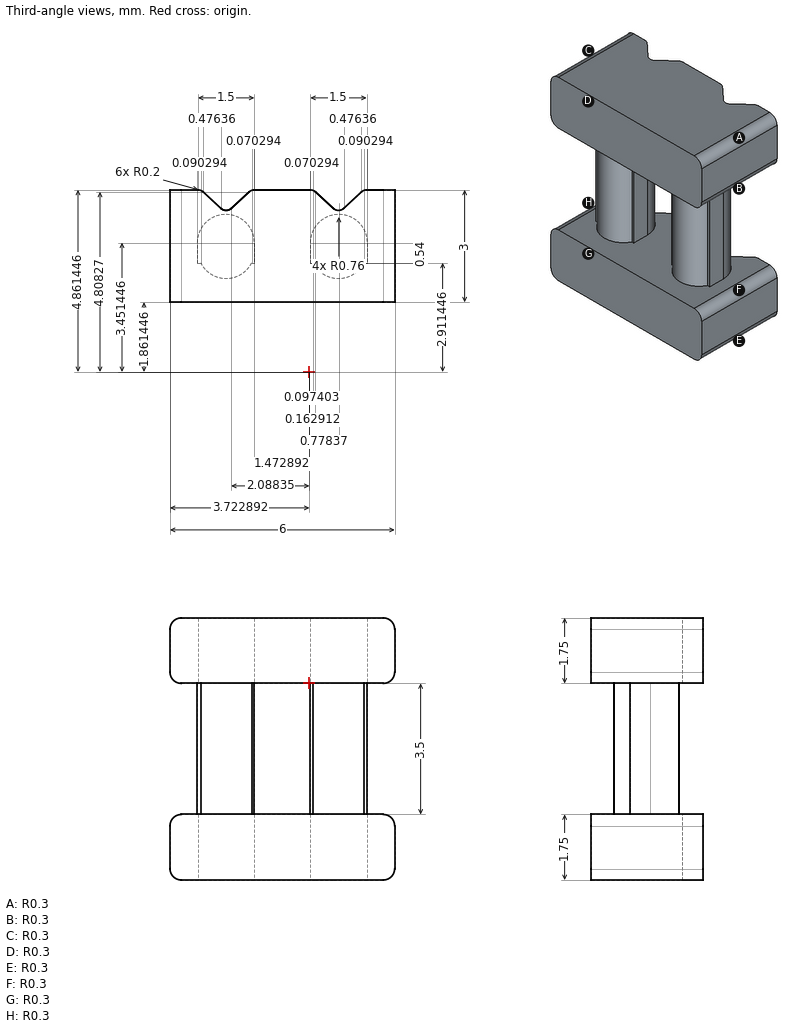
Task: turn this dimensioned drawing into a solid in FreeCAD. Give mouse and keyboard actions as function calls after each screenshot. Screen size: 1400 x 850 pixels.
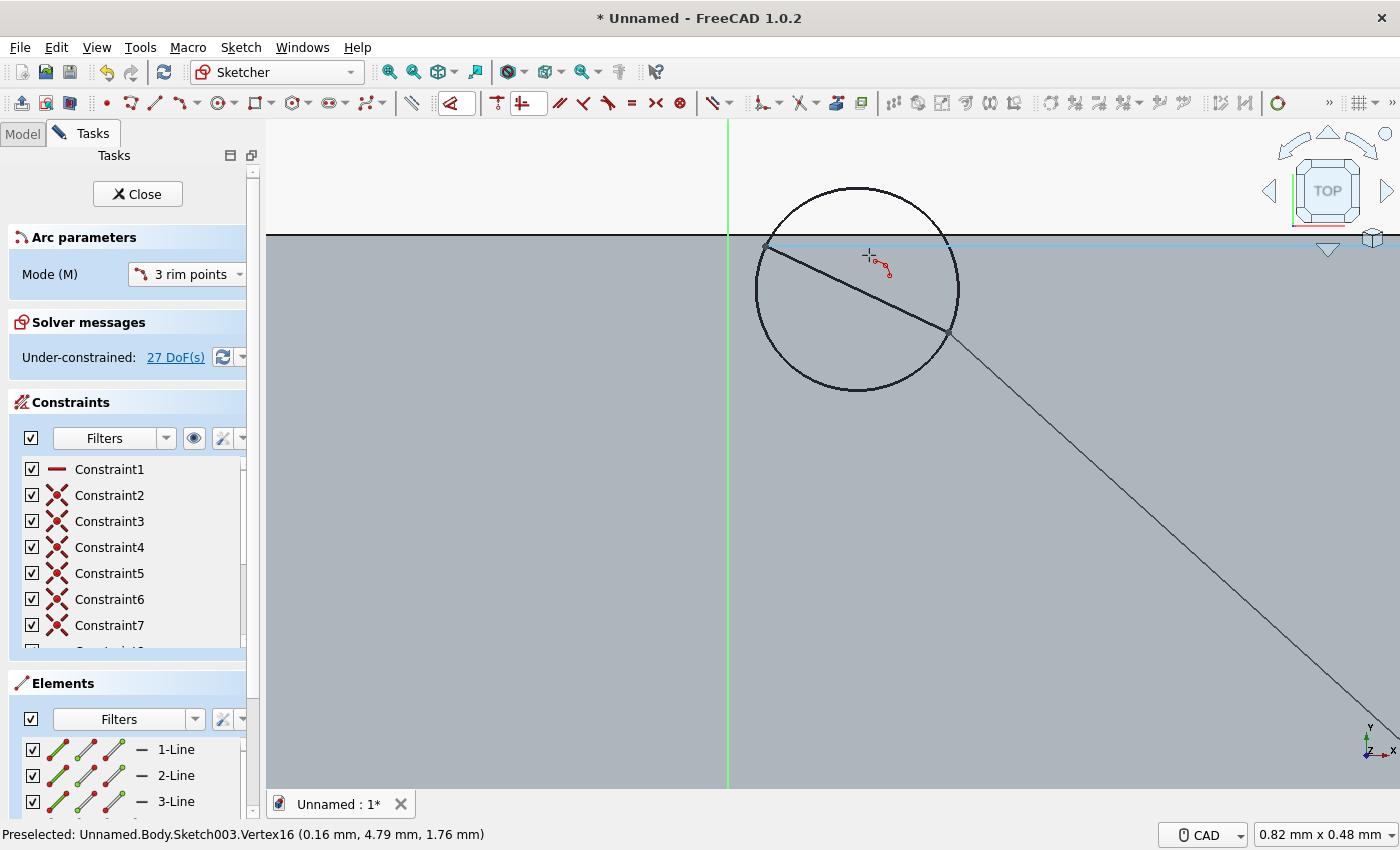
click(867, 254)
key(Escape)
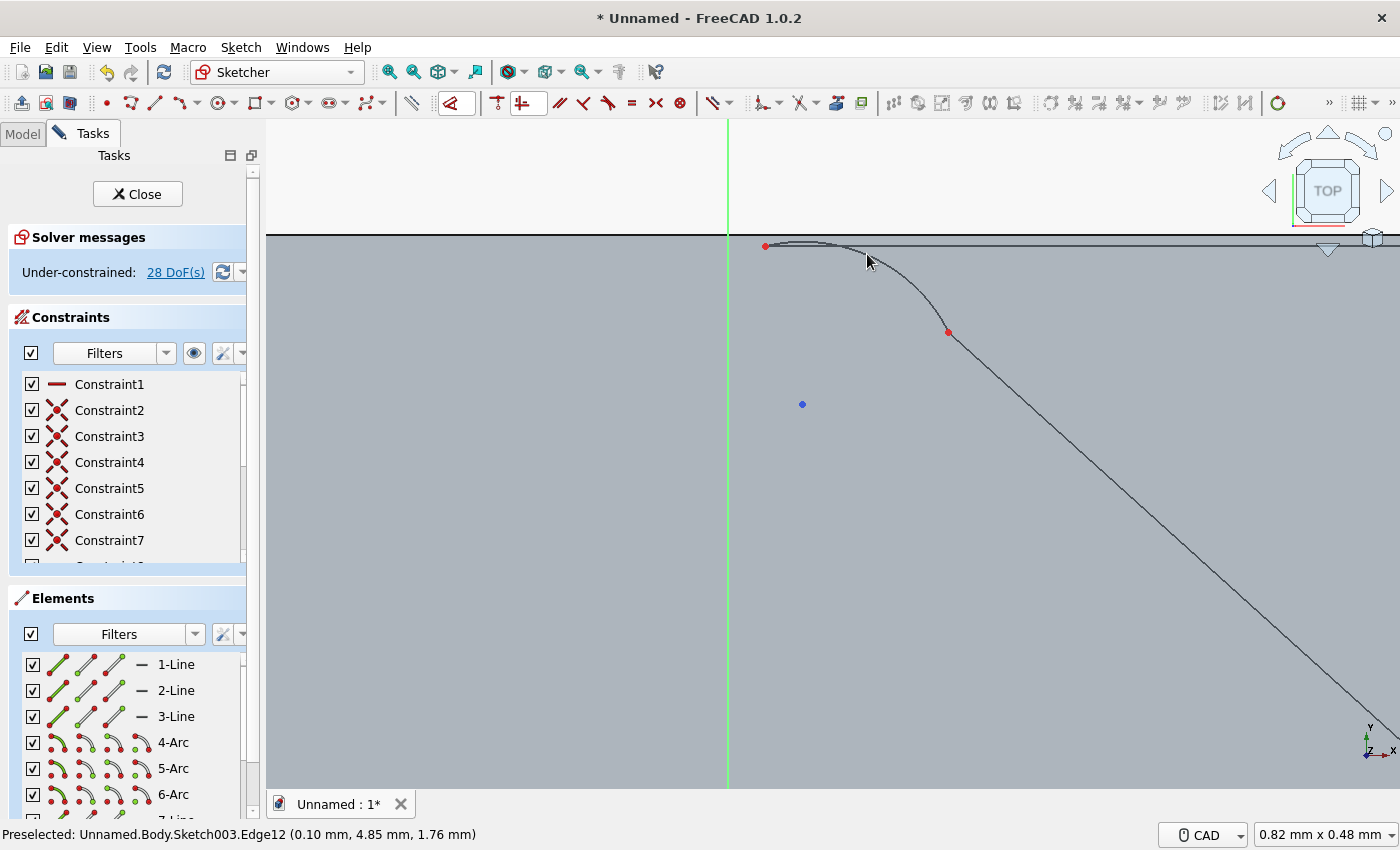
scroll(832, 250, down, 14)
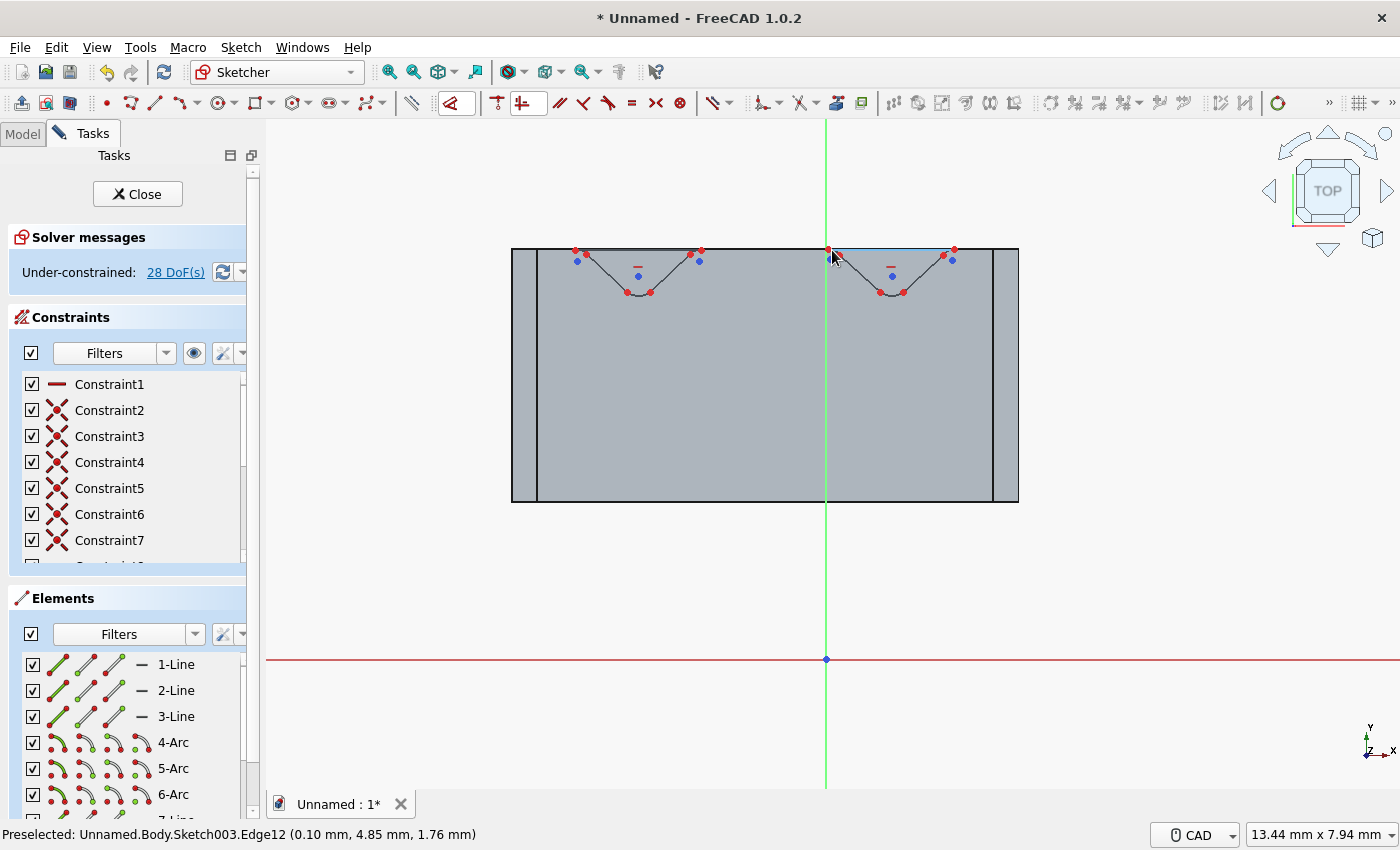
click(664, 250)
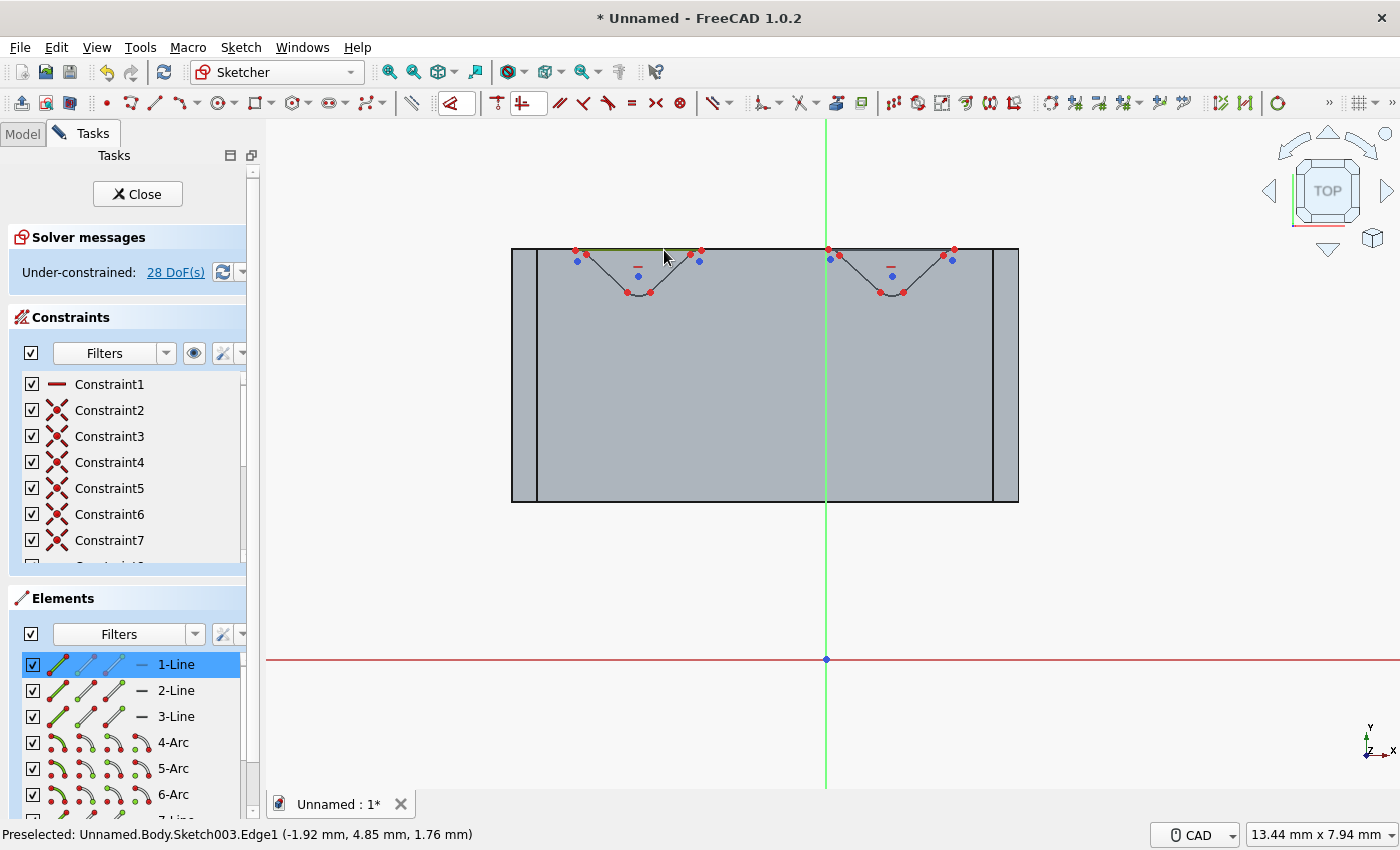
scroll(585, 252, up, 9)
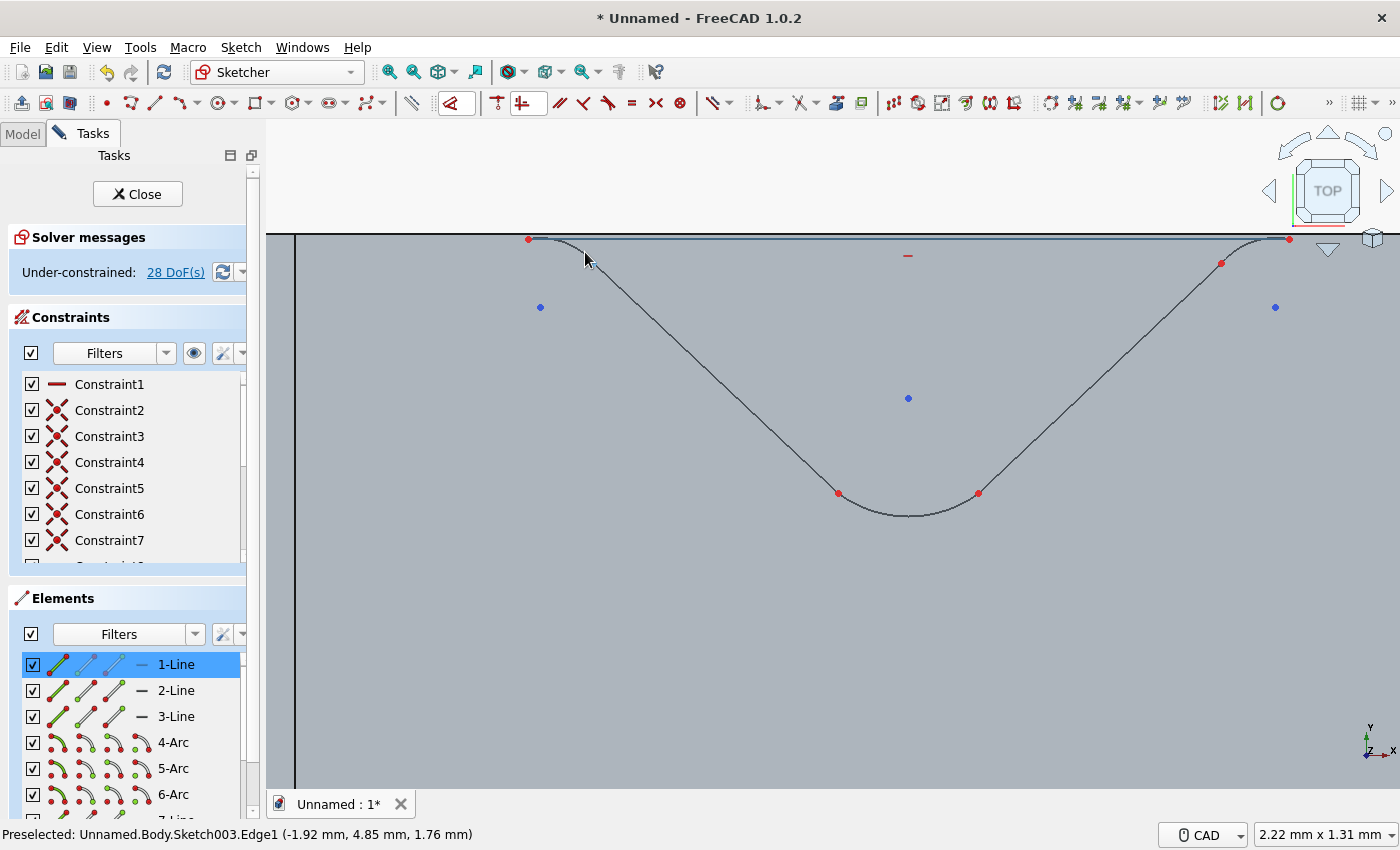
click(583, 253)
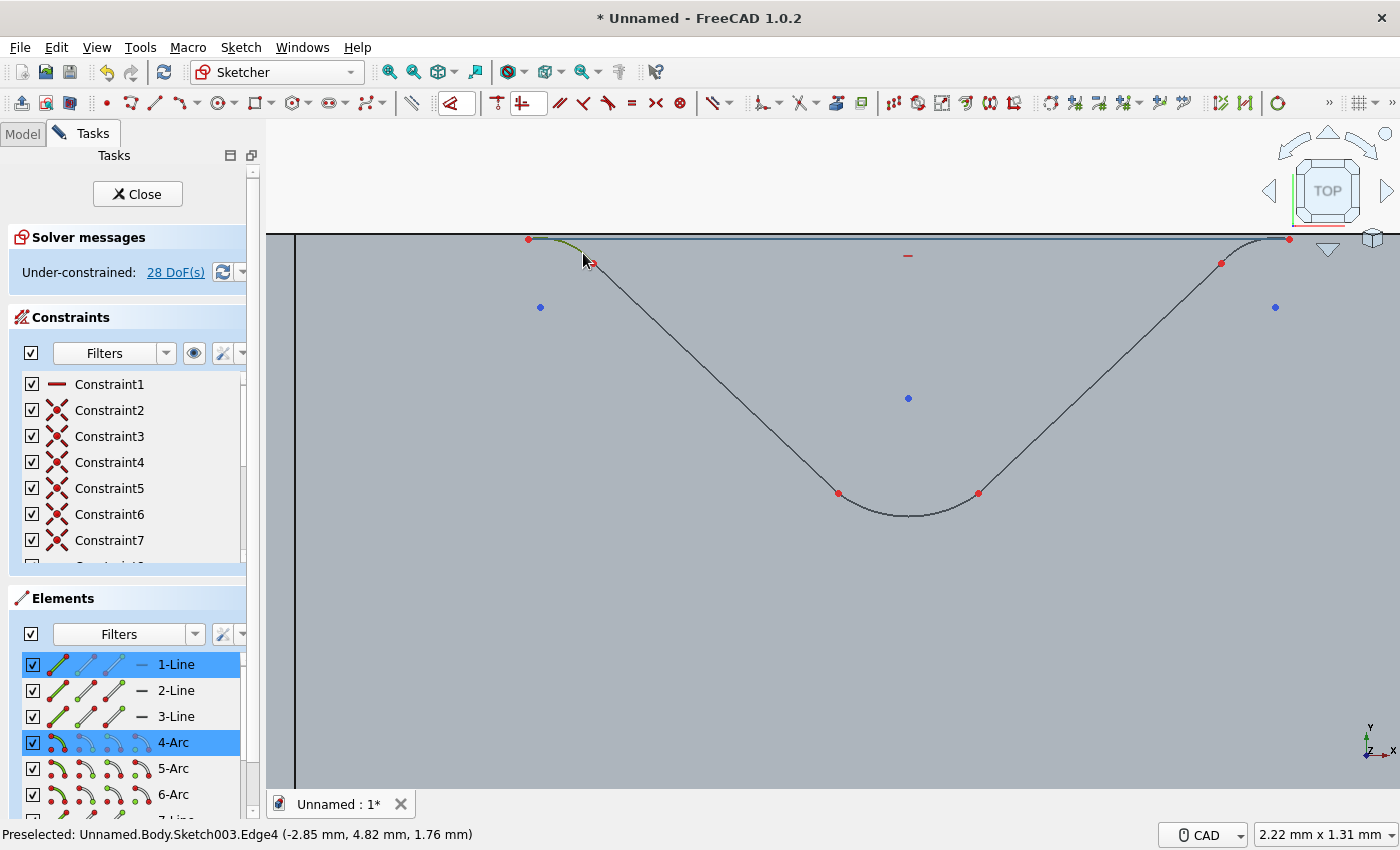
click(608, 104)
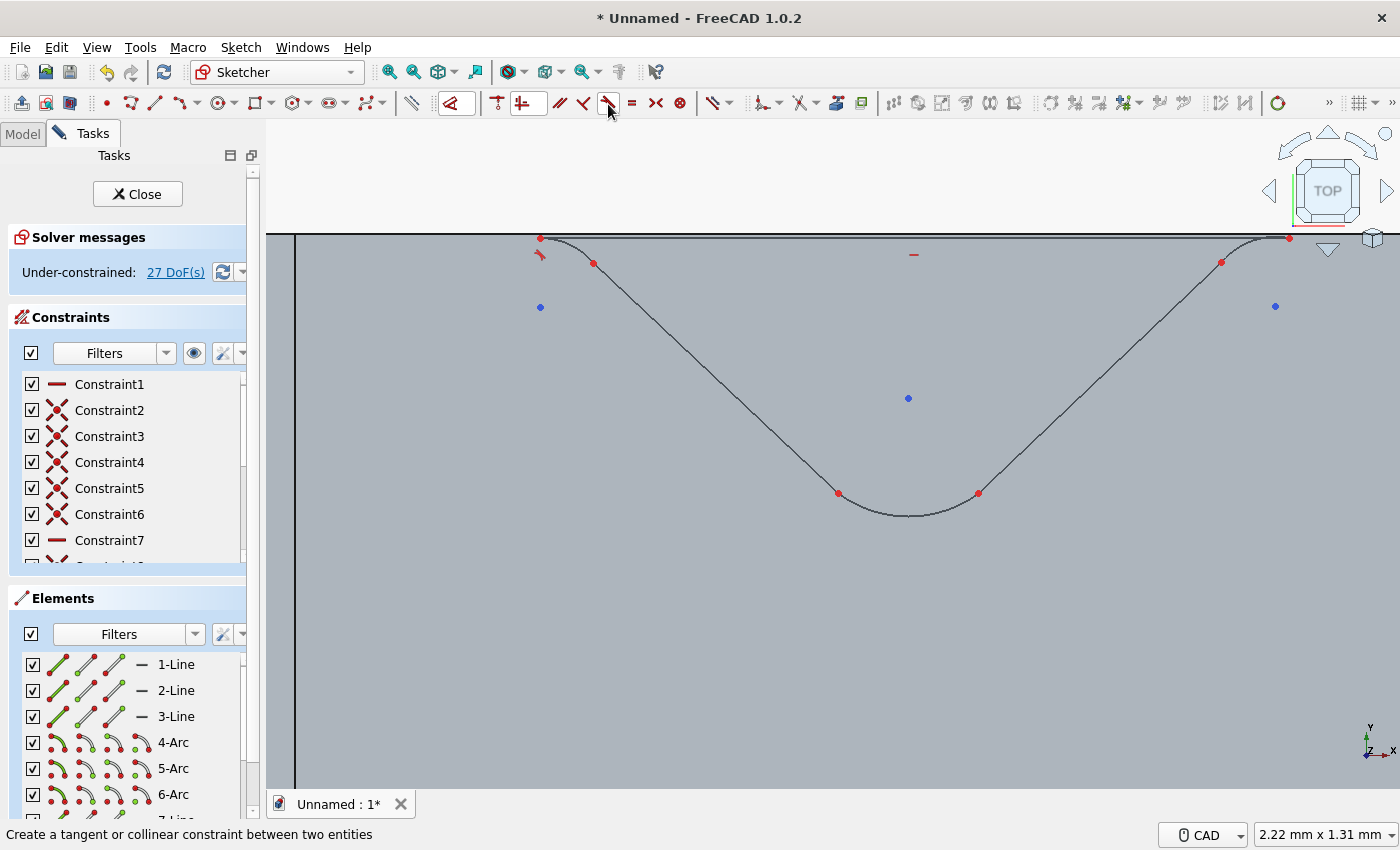
scroll(584, 252, down, 9)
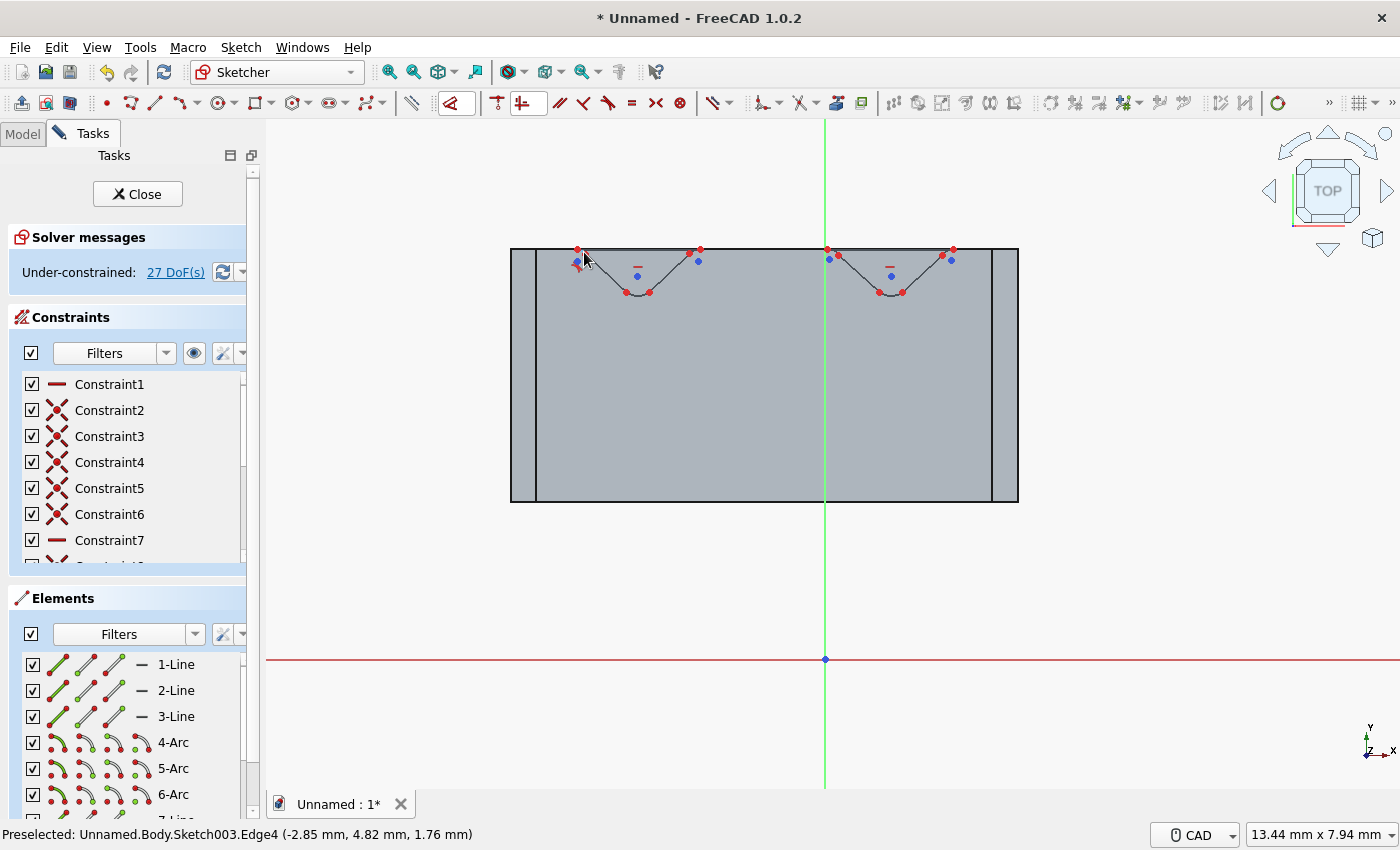
click(664, 250)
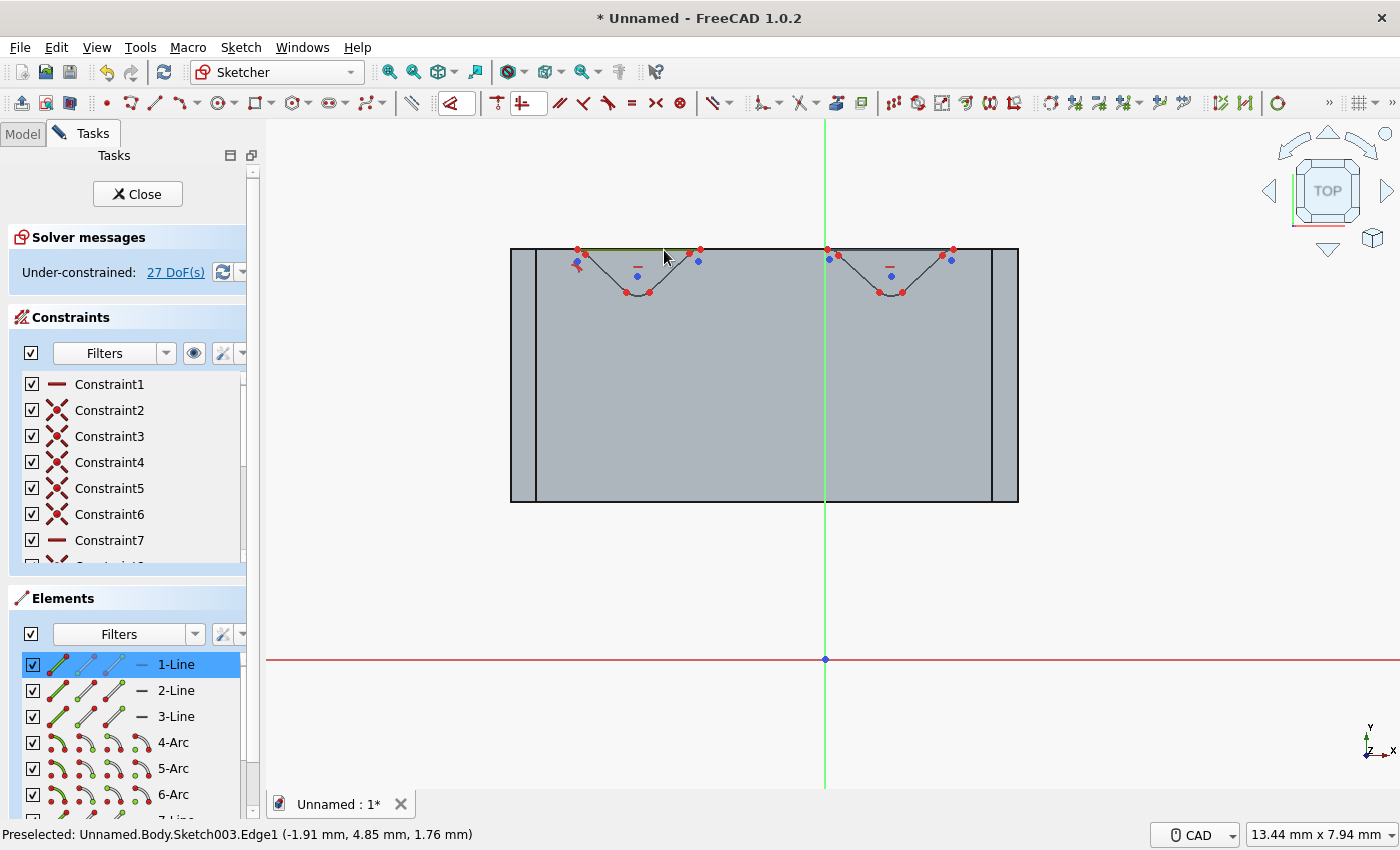
scroll(691, 252, up, 10)